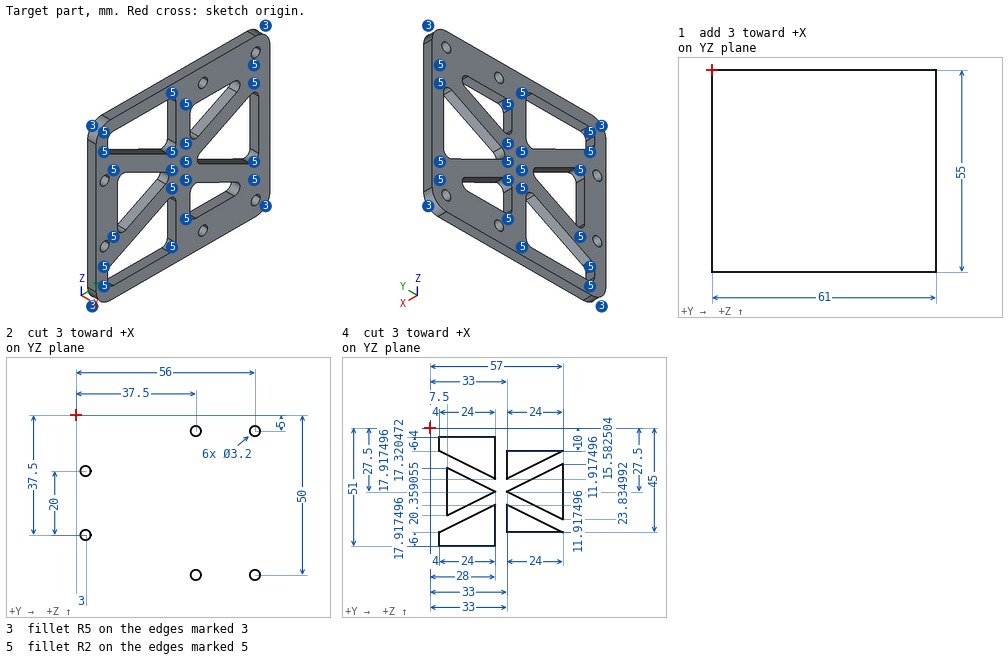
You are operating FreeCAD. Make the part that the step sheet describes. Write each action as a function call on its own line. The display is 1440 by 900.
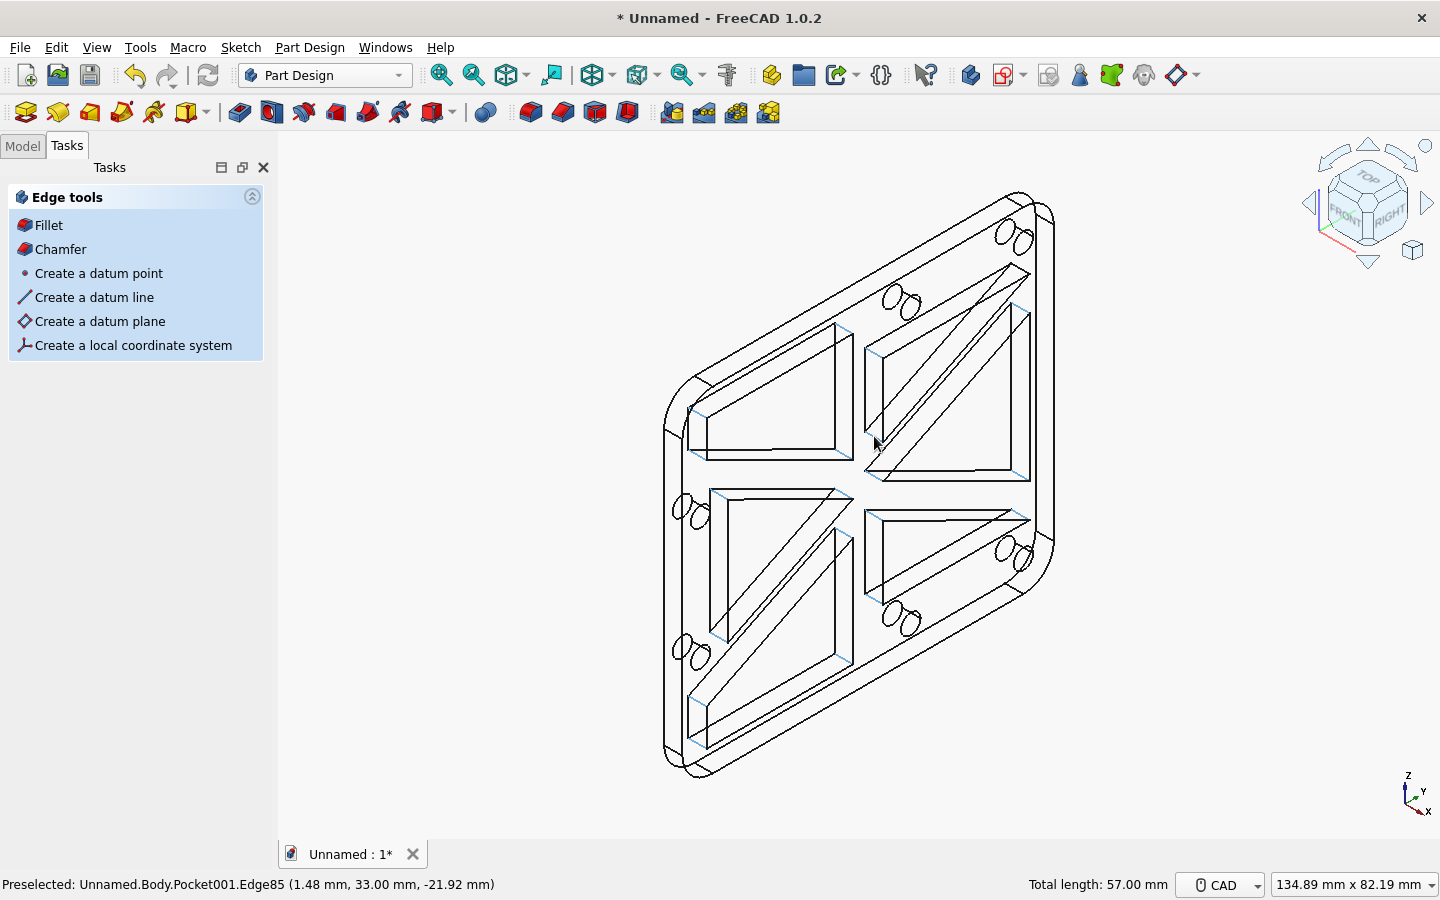
click(1020, 268, ctrl)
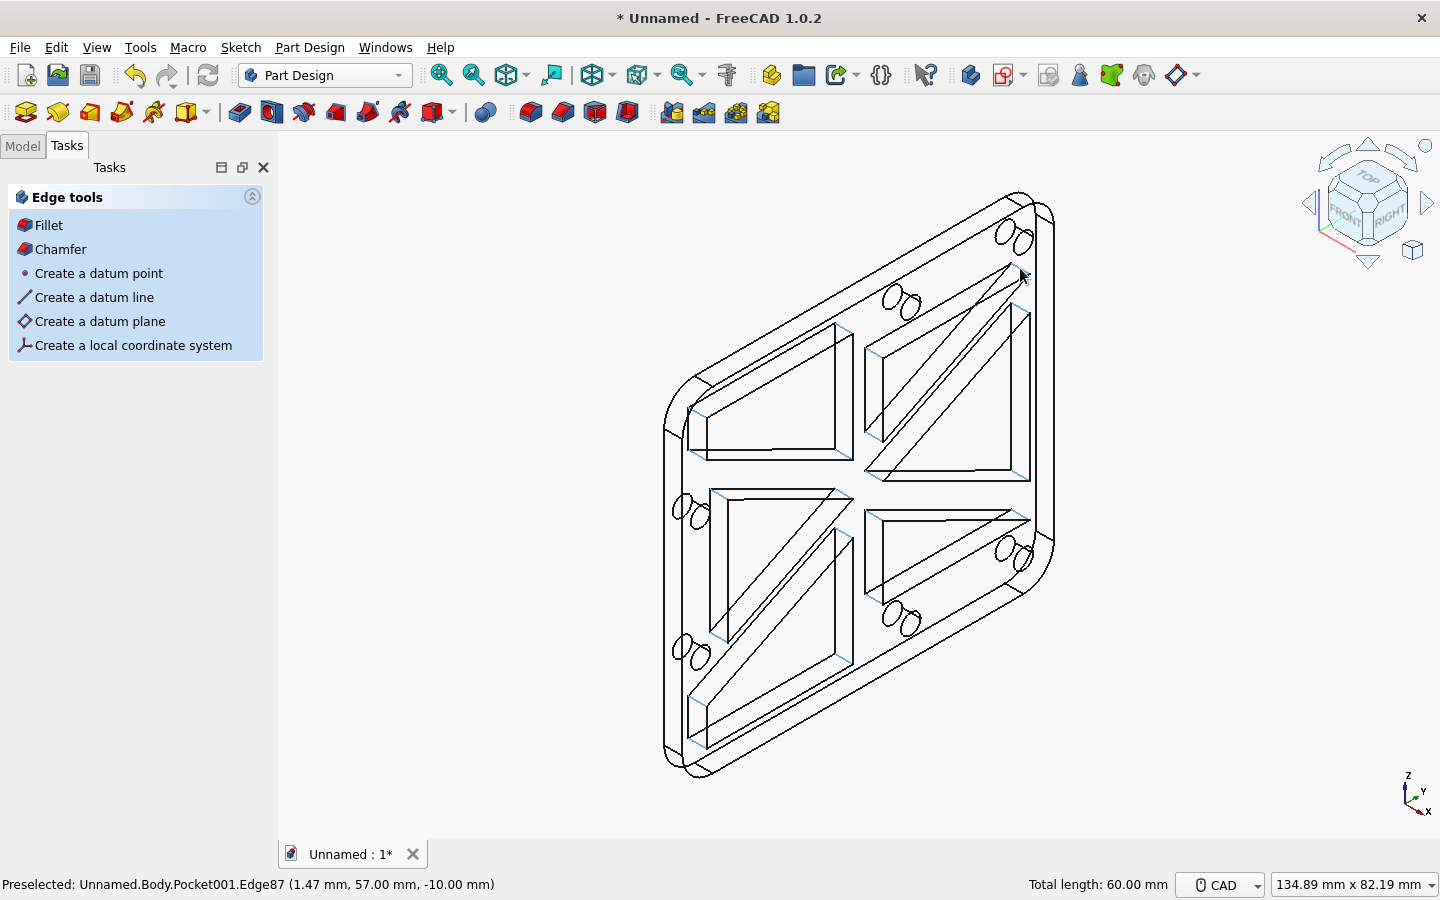
key(v)
key(1)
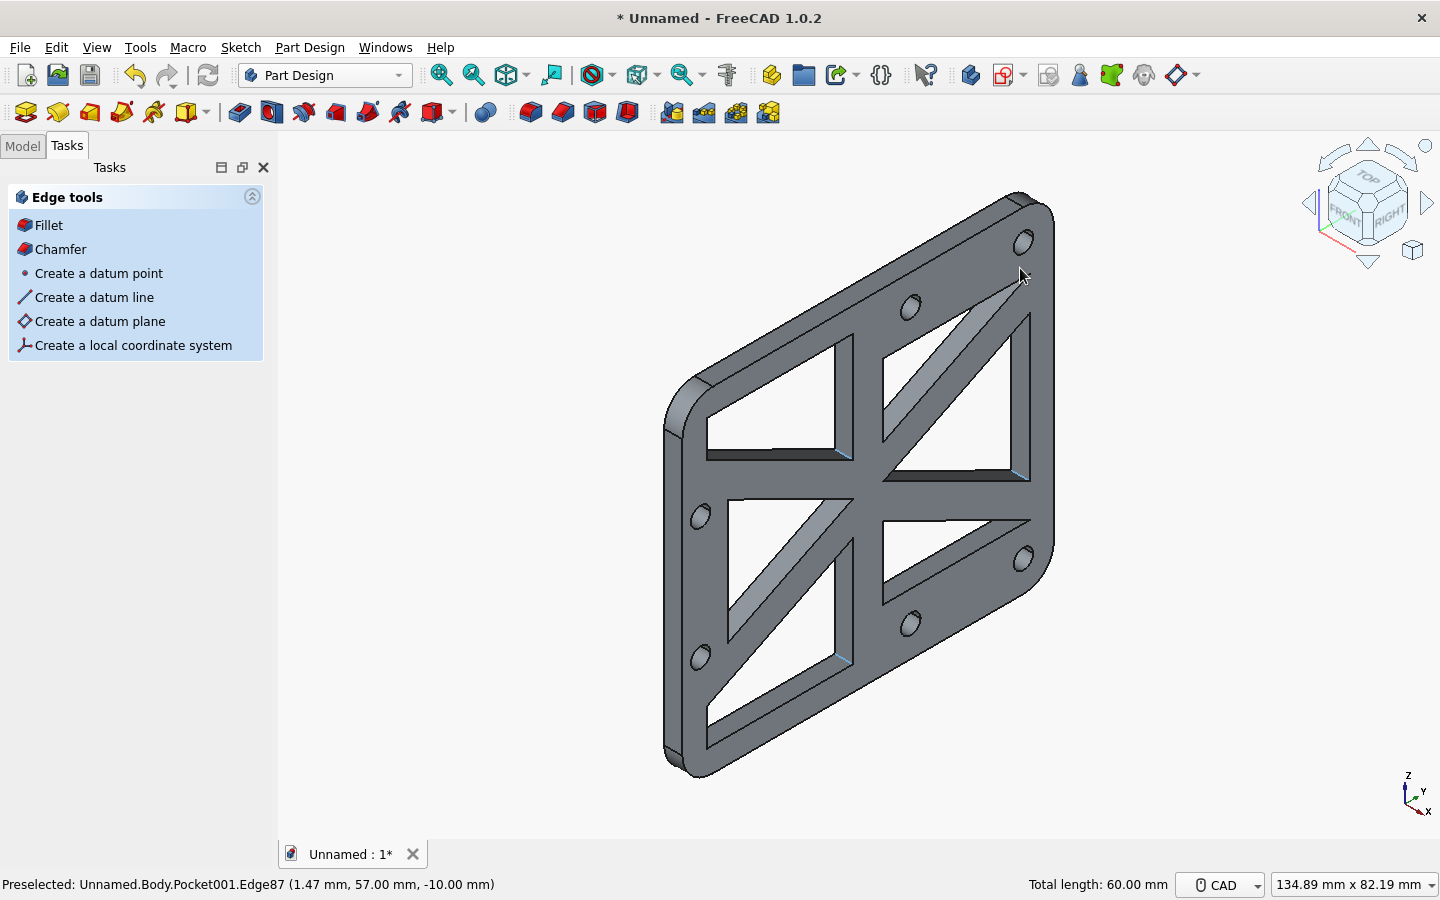
click(532, 112)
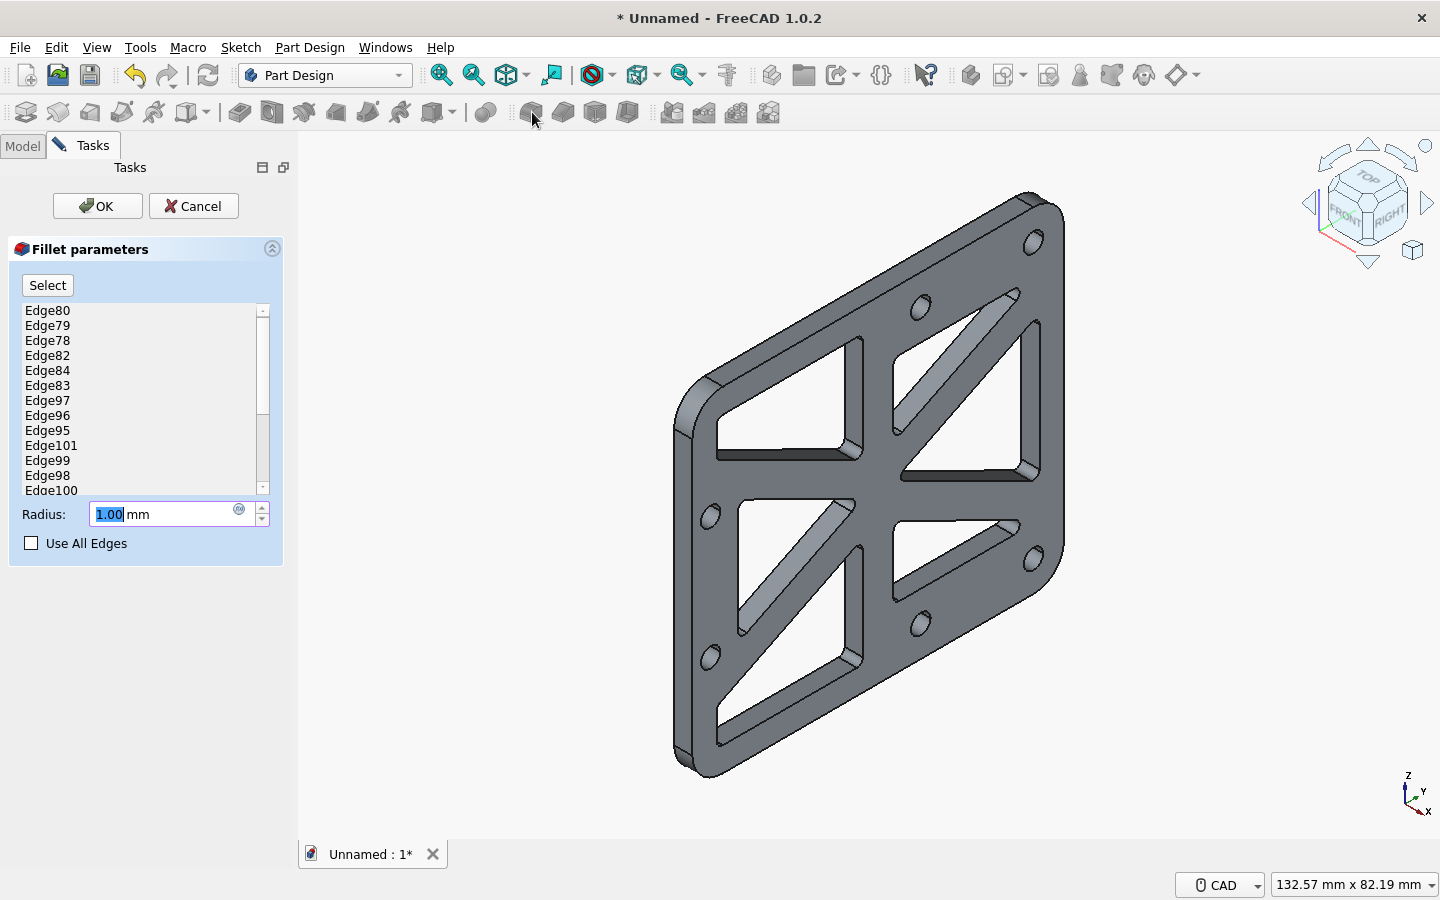
text(2)
key(Tab)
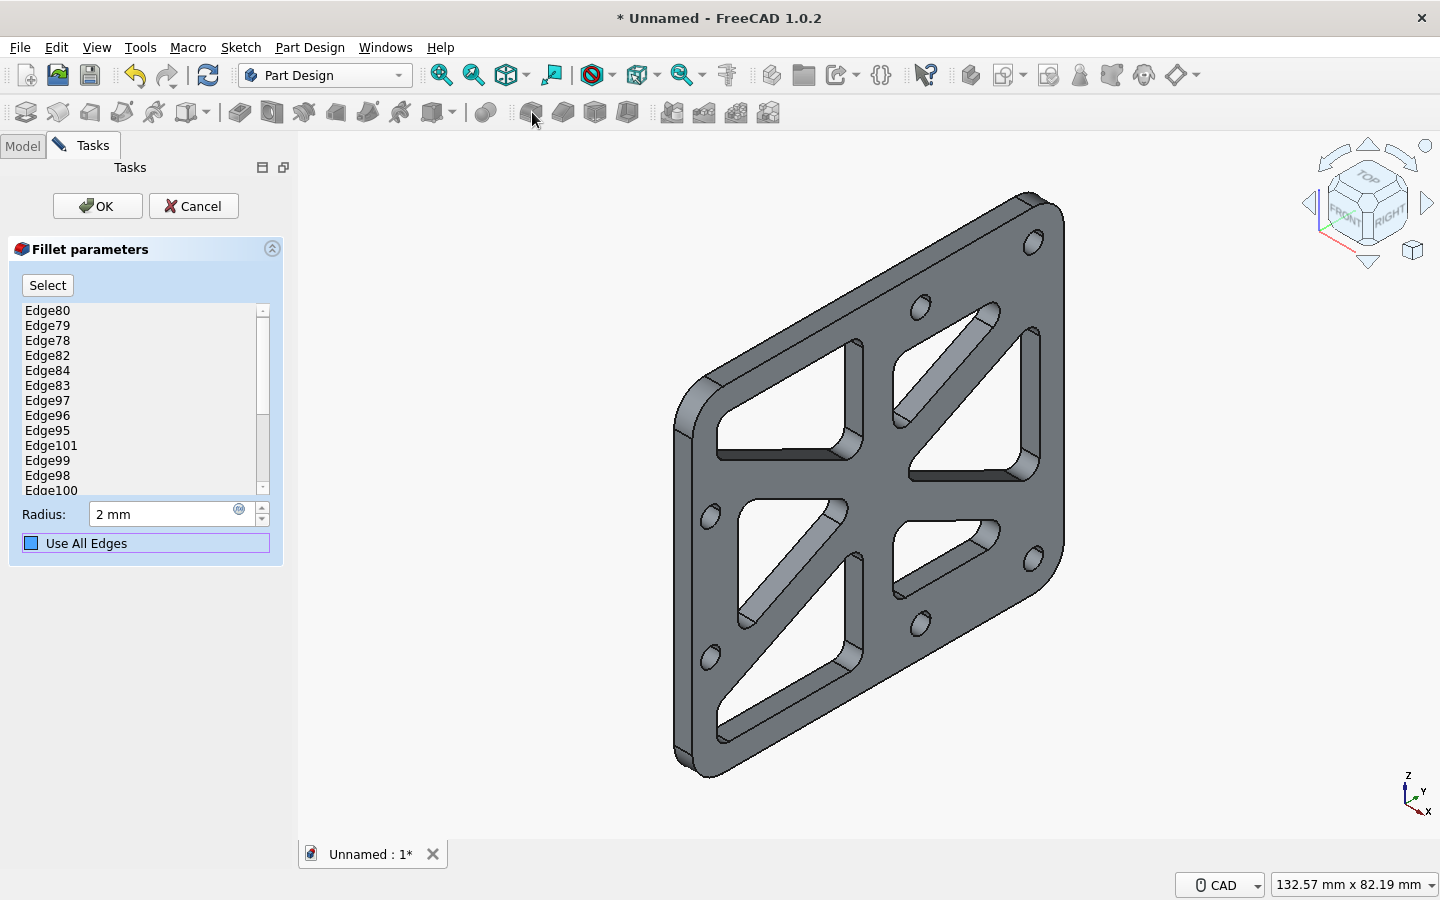
click(98, 206)